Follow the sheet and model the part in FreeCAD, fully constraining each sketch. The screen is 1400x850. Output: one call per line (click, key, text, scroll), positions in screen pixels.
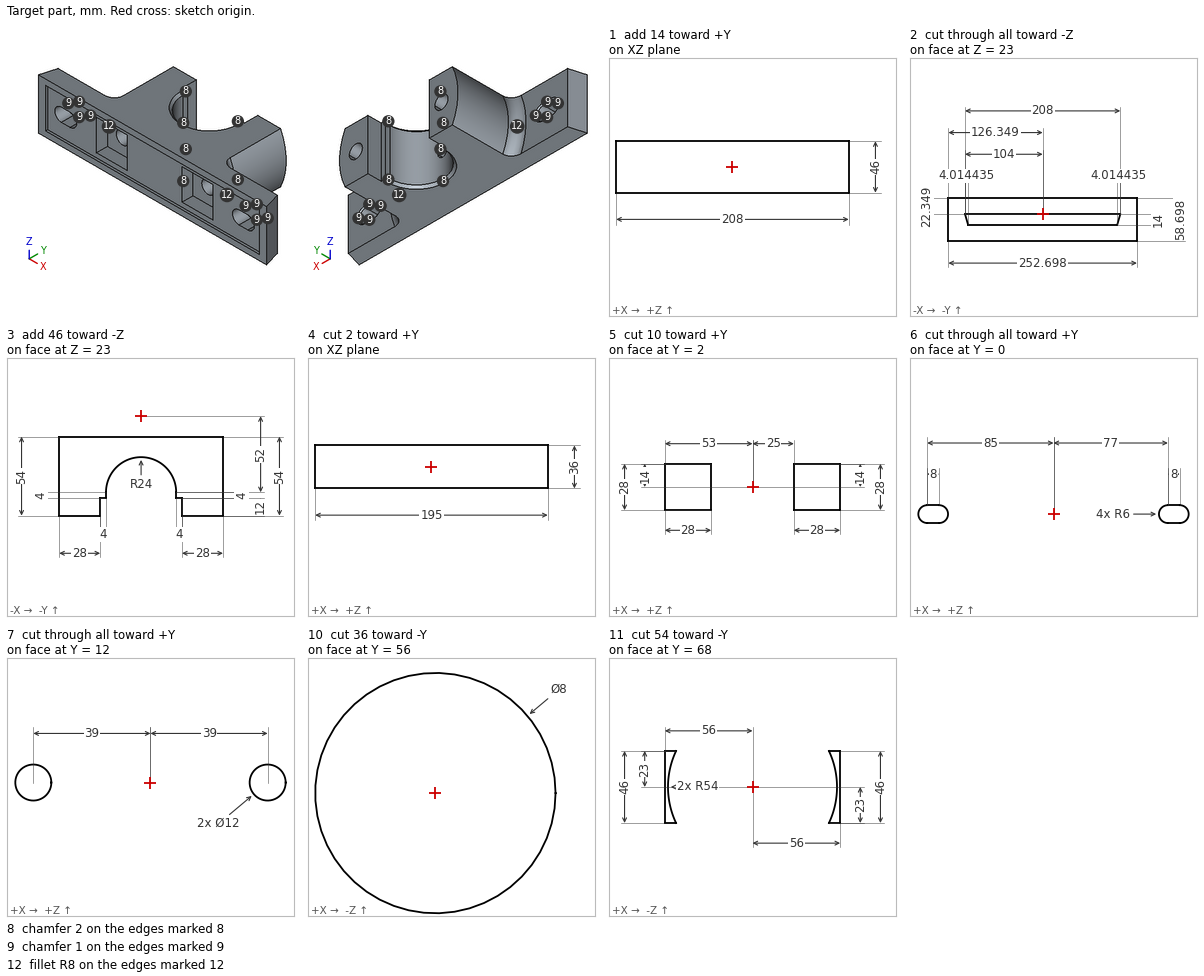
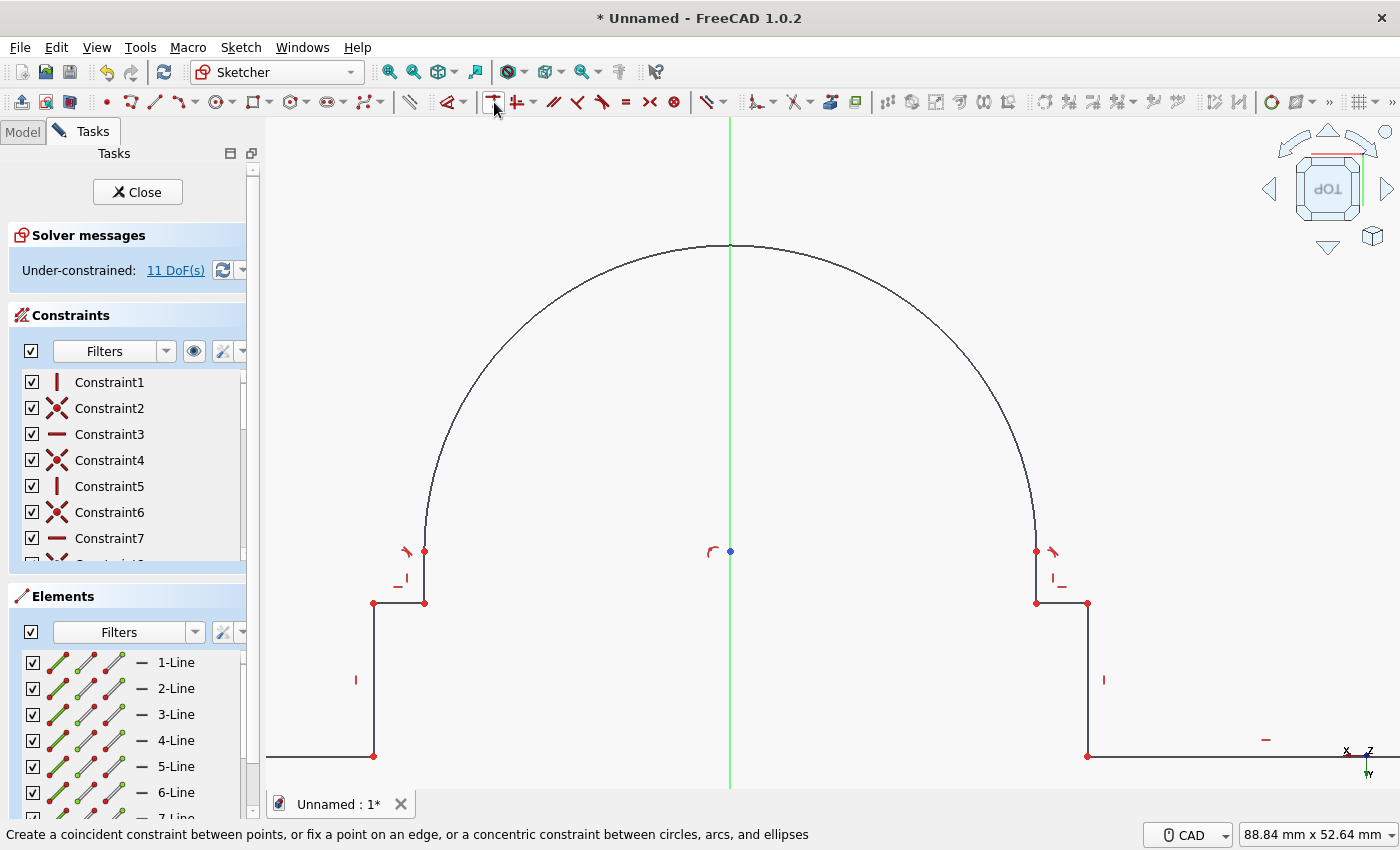
click(910, 304)
click(929, 278)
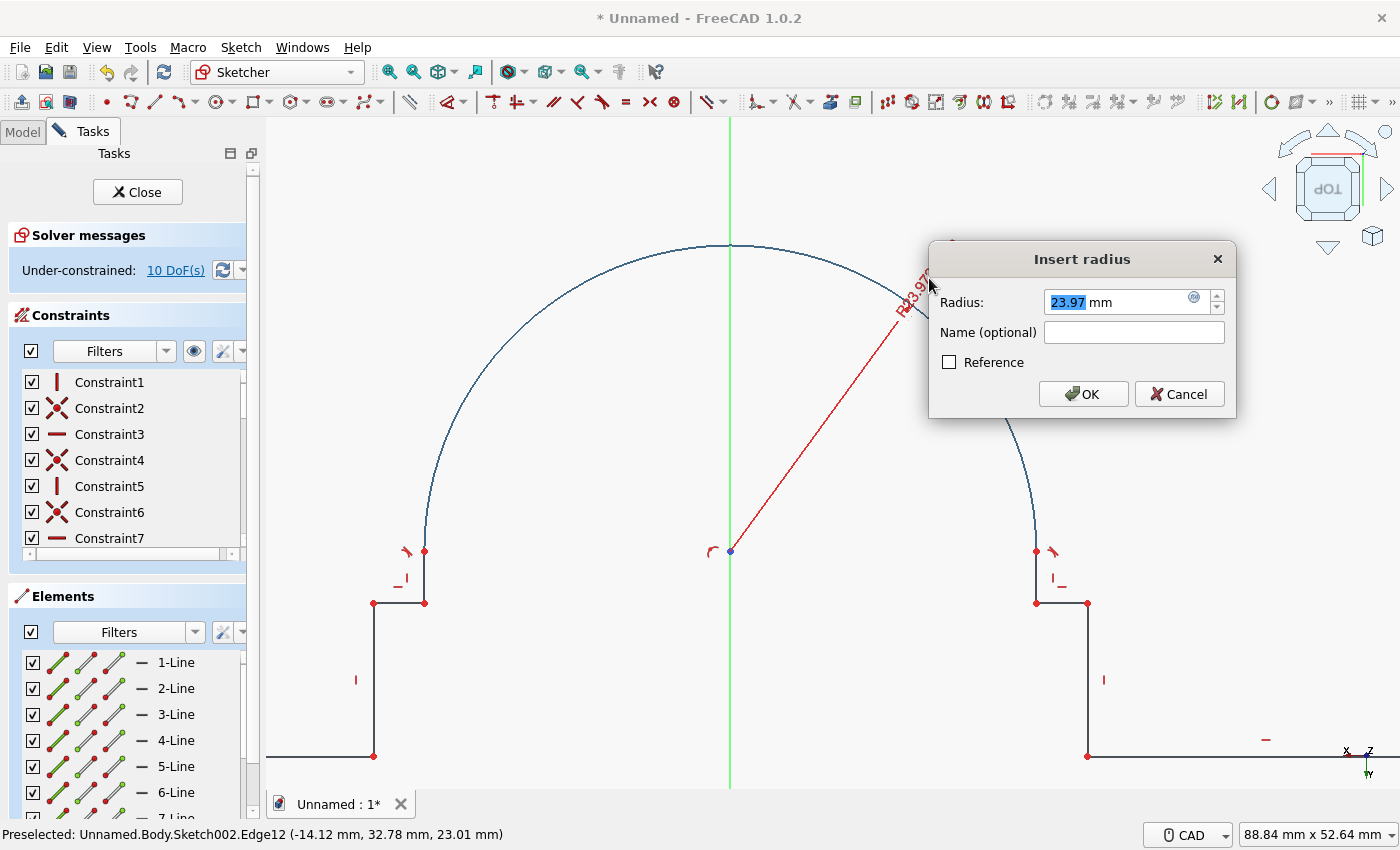
text(24)
key(Return)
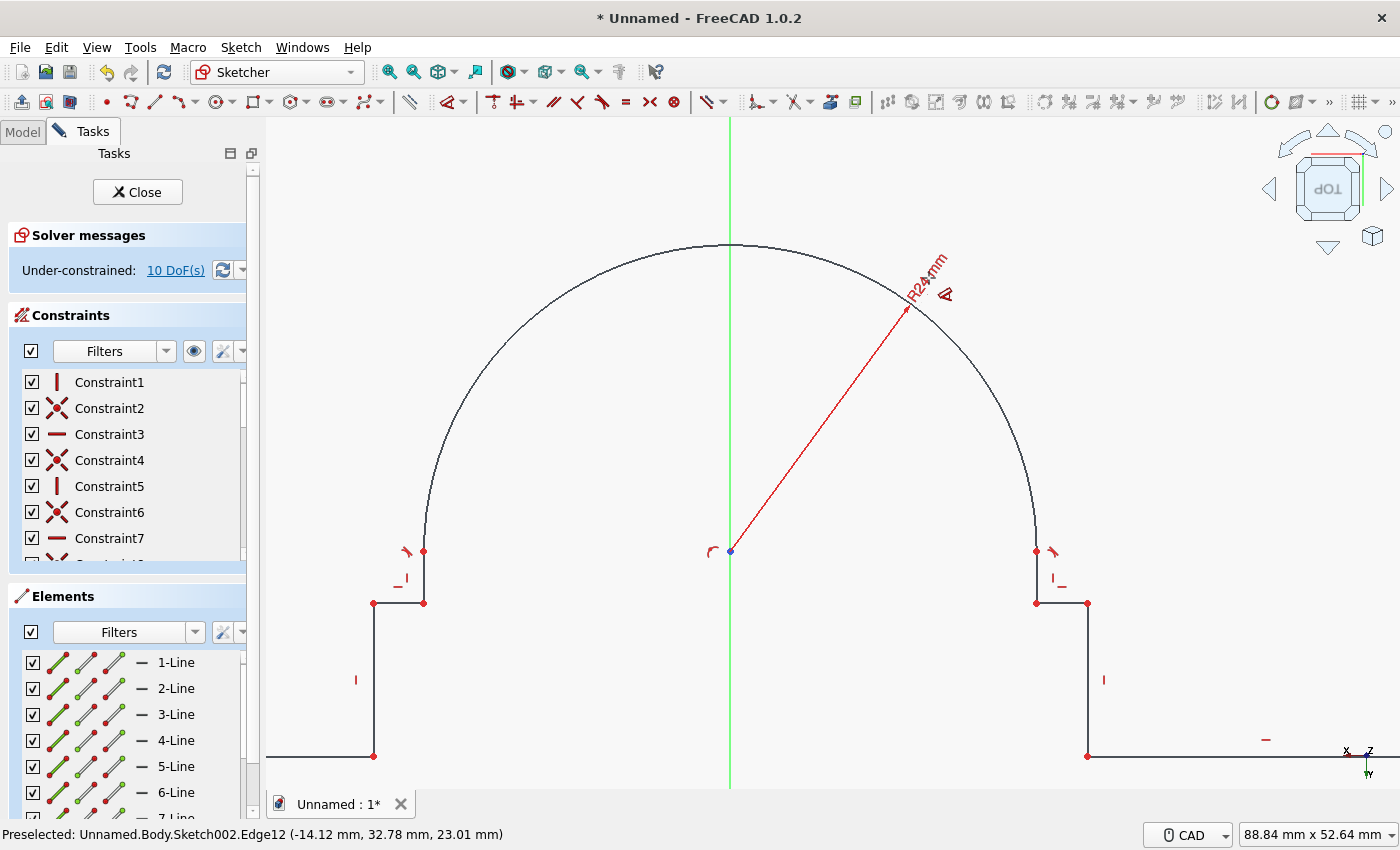
click(1037, 567)
click(1071, 577)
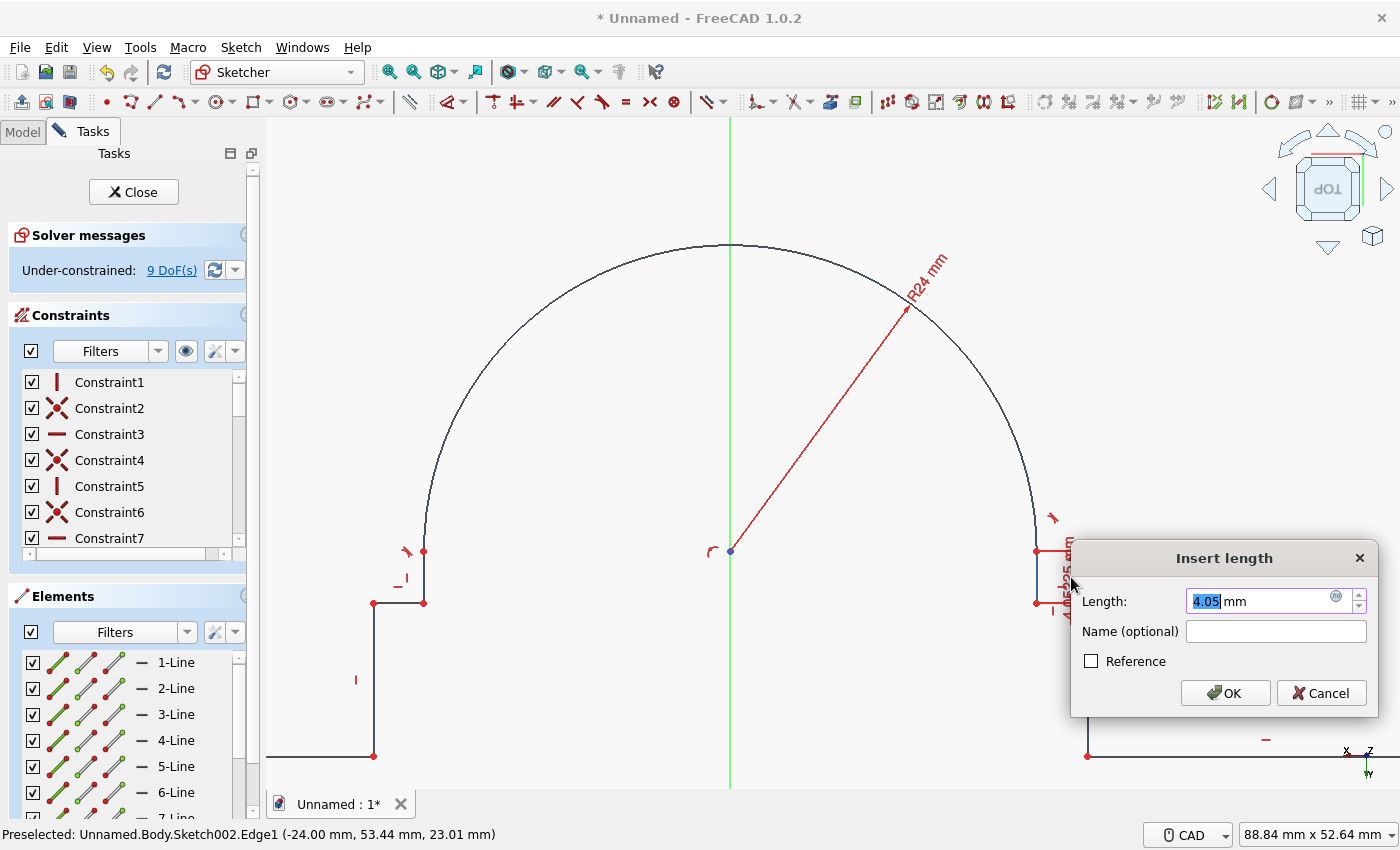
text(4)
key(Return)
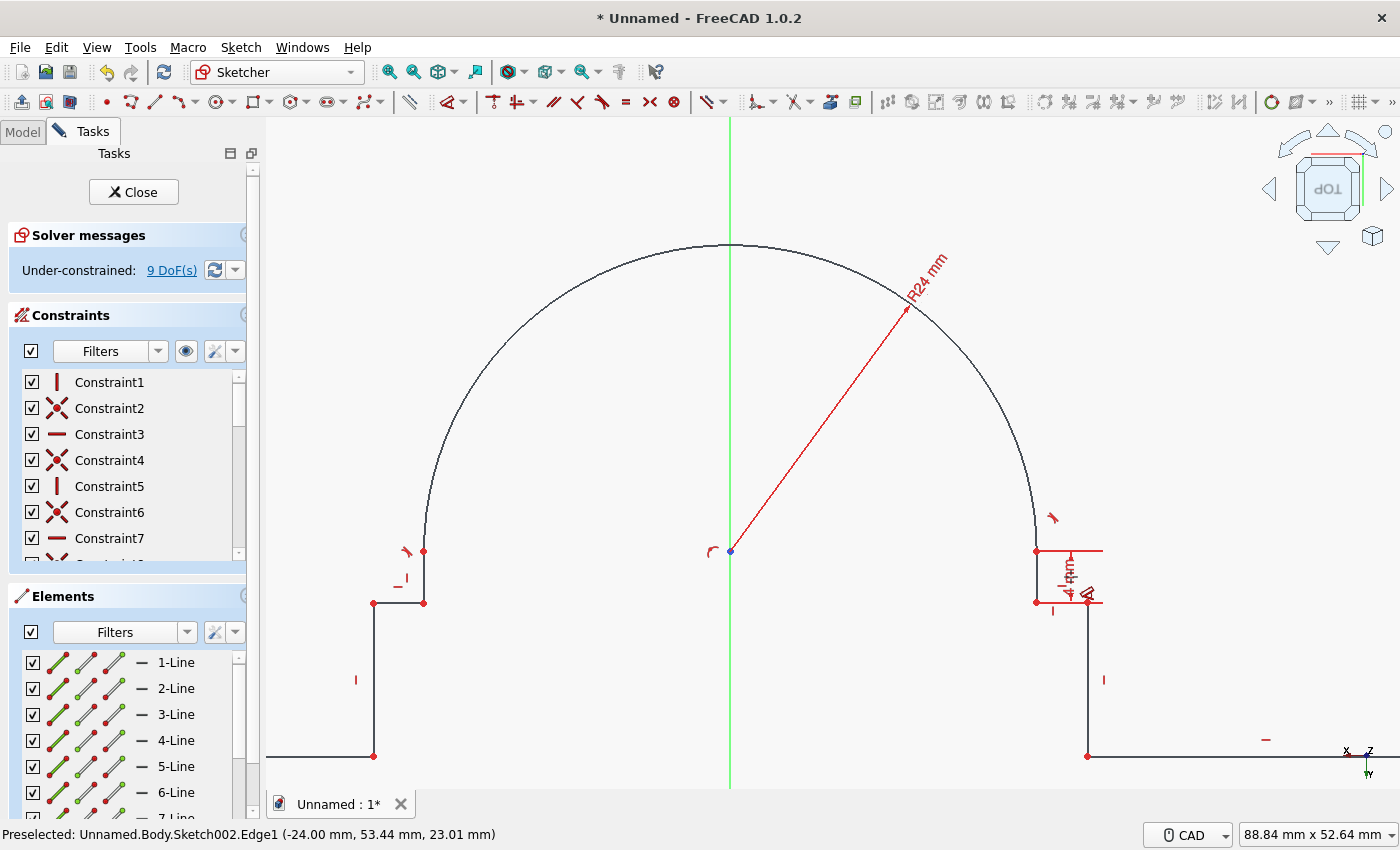
click(1052, 603)
click(1062, 637)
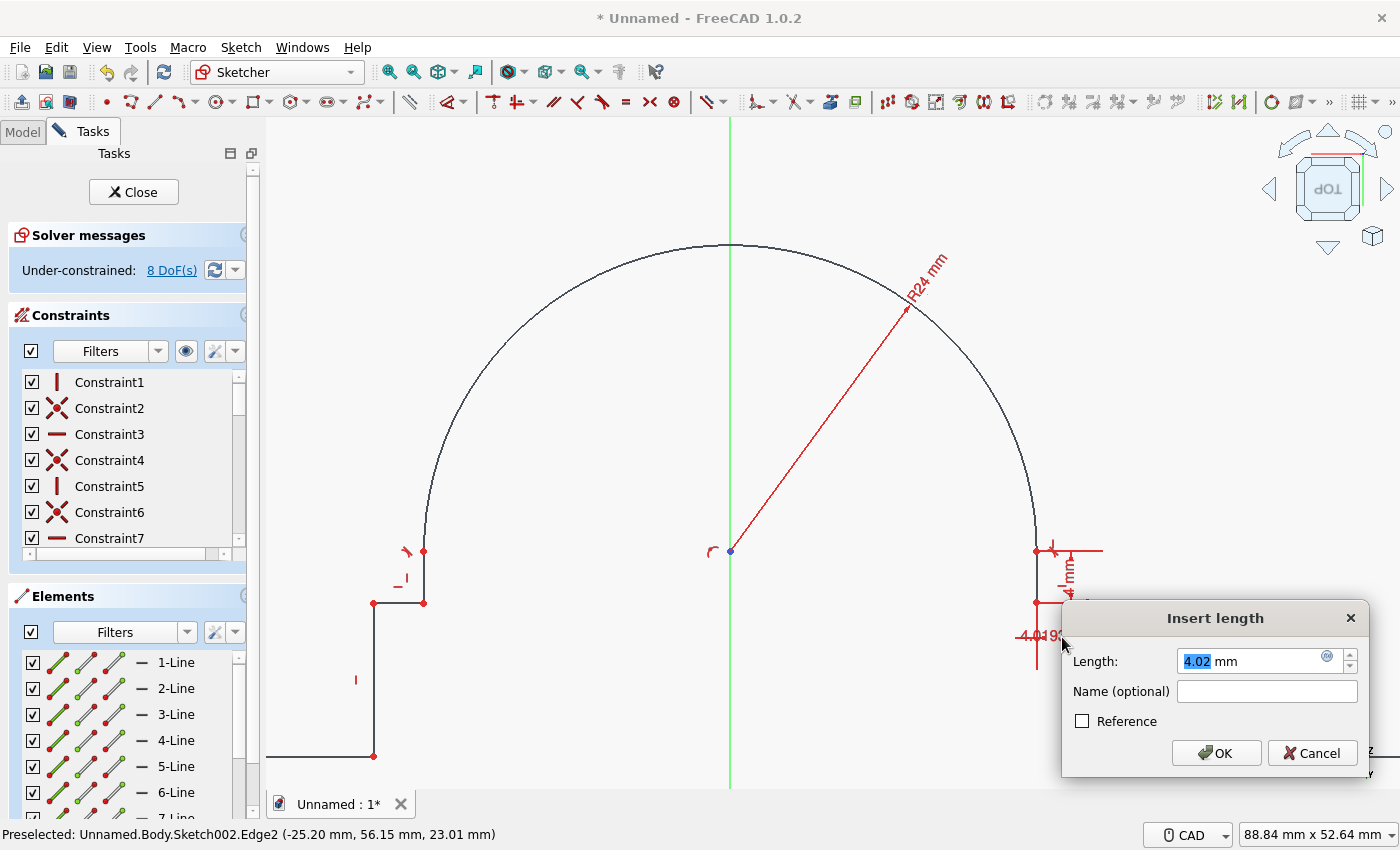
text(4)
key(Return)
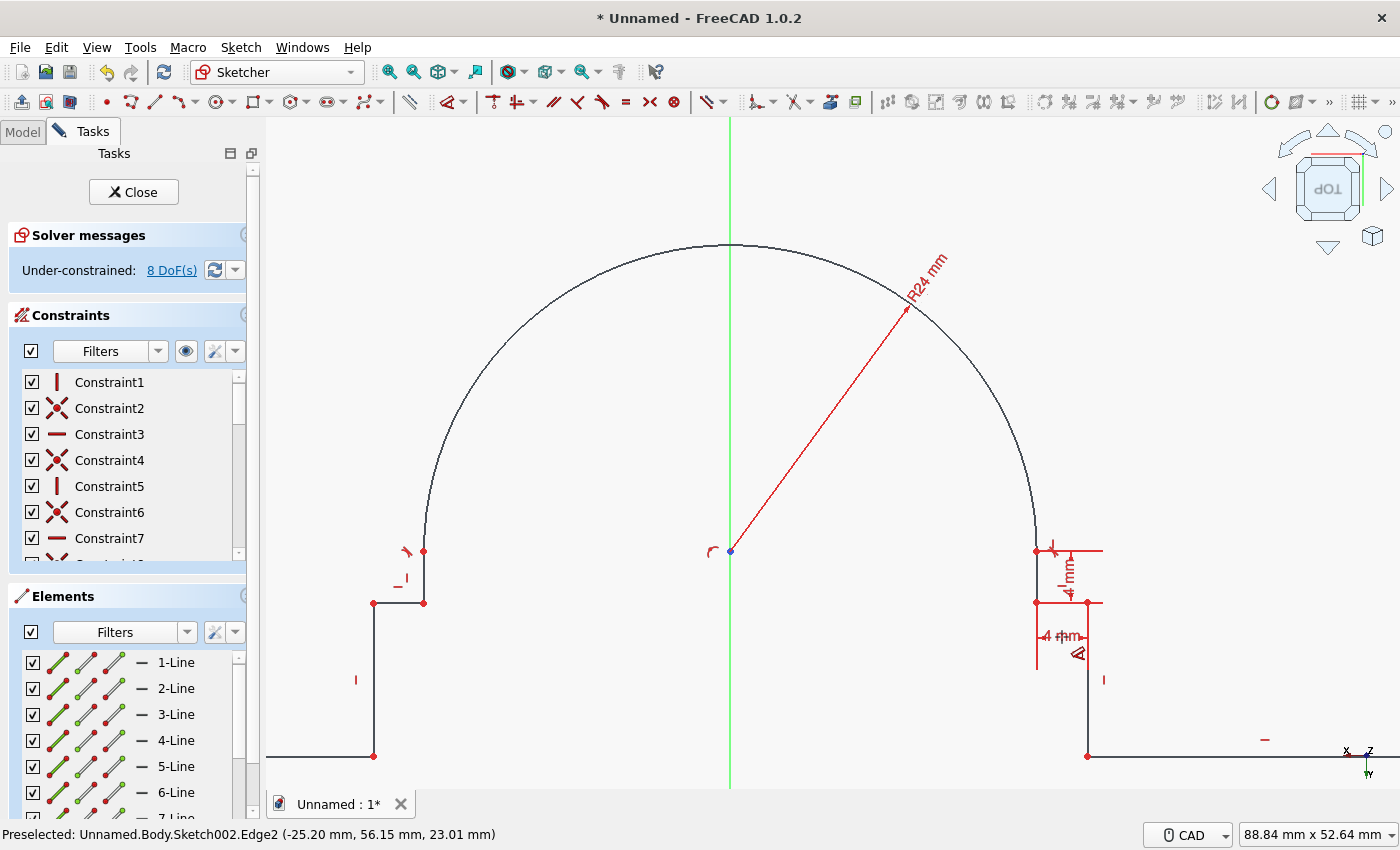
click(389, 603)
click(399, 637)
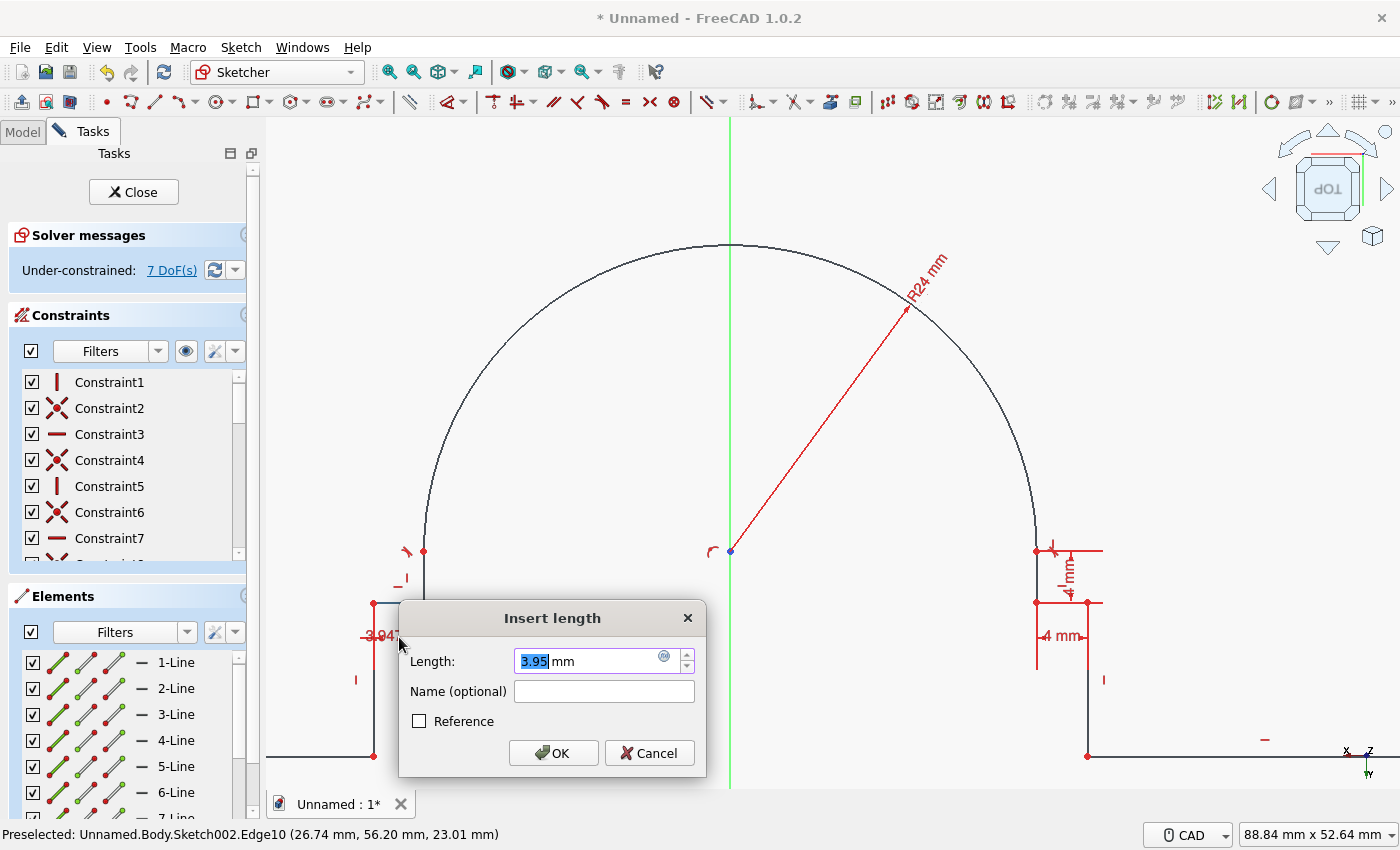
text(4)
key(Return)